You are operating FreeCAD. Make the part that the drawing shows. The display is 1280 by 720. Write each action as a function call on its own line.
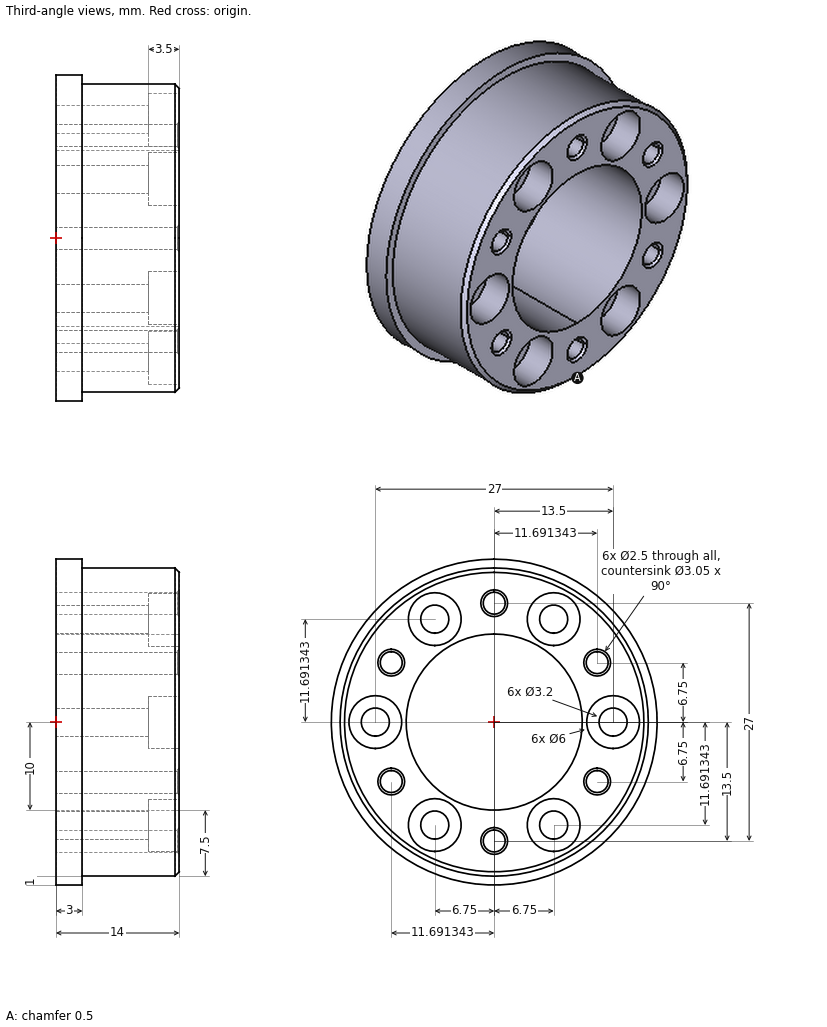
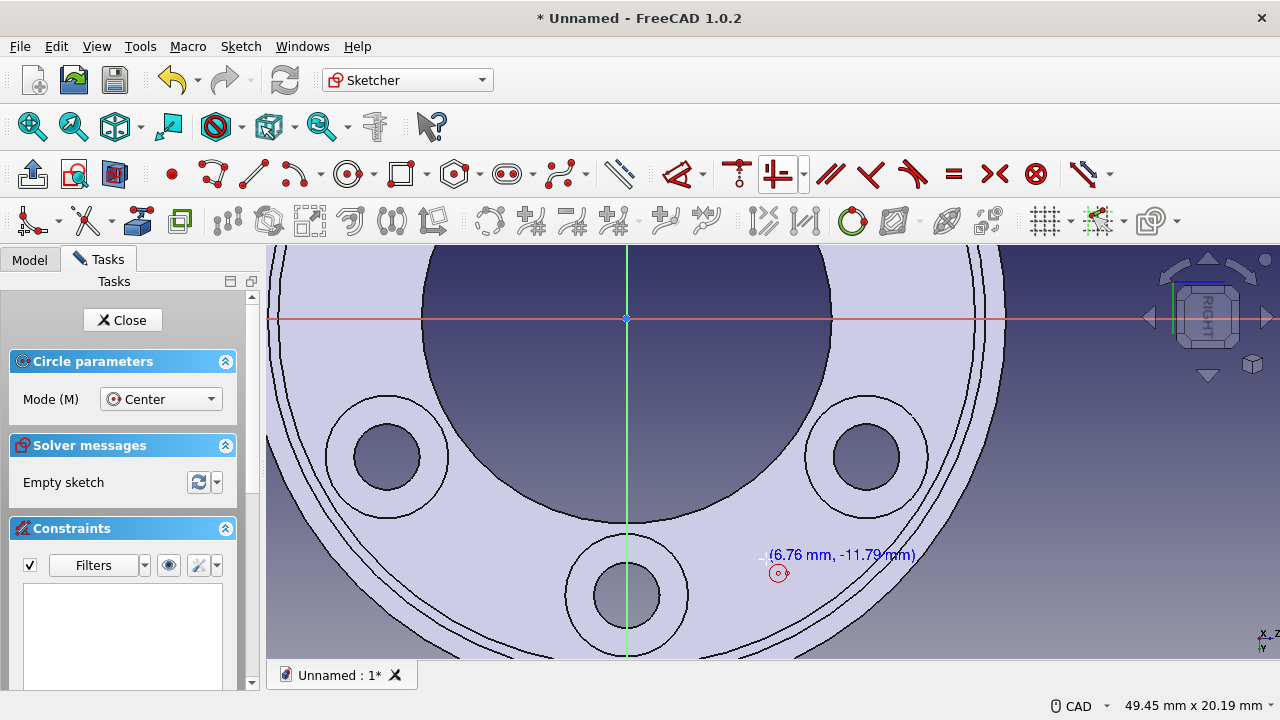
click(765, 558)
click(783, 540)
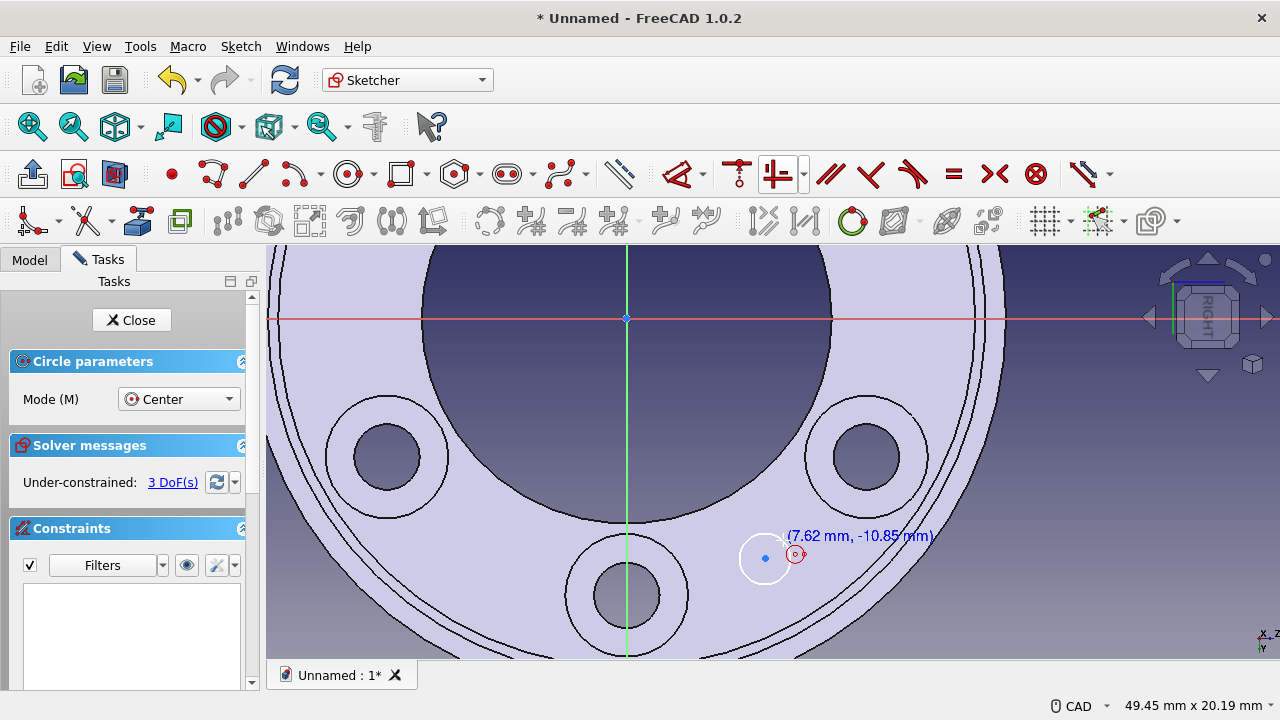
click(488, 558)
click(506, 540)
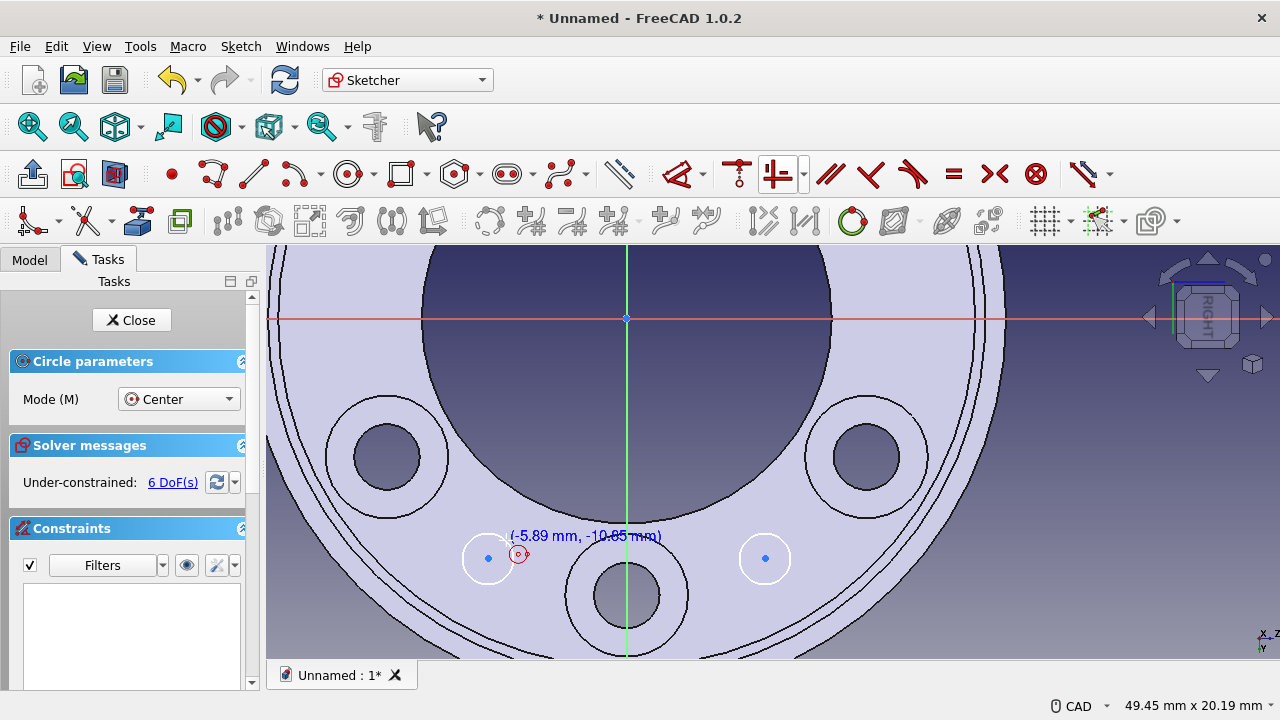
click(350, 319)
click(368, 300)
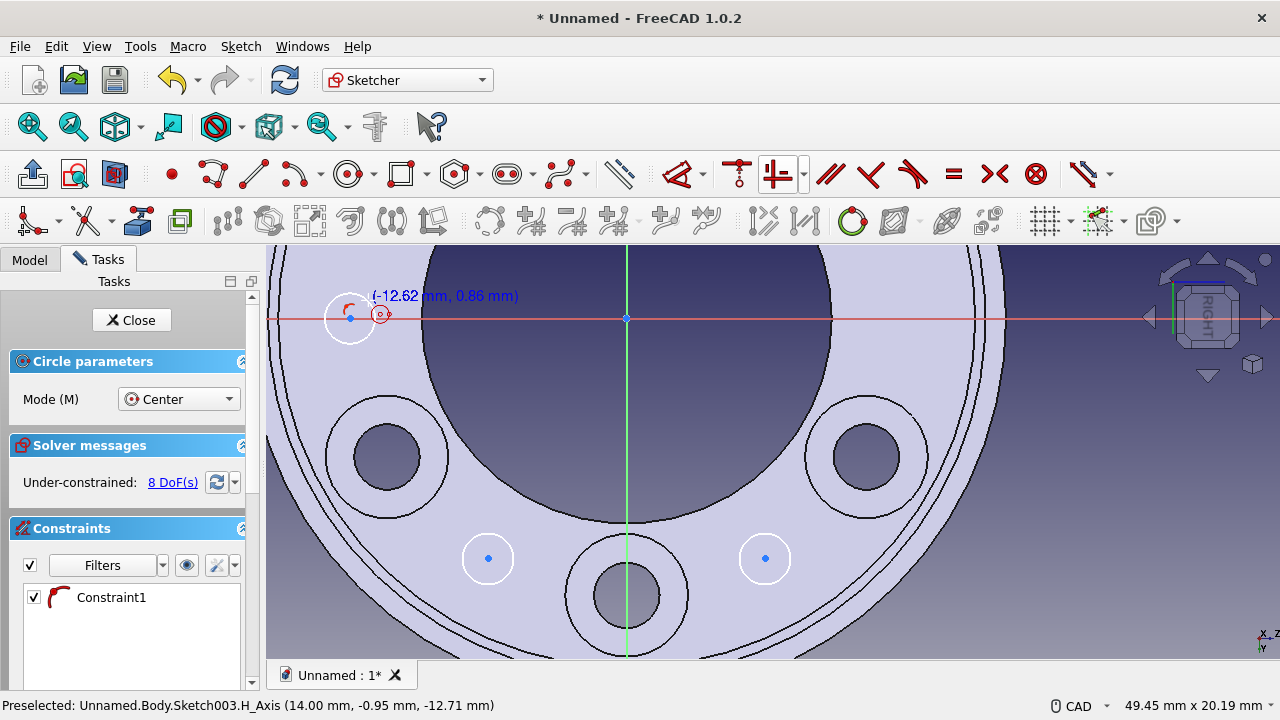
scroll(768, 561, down, 4)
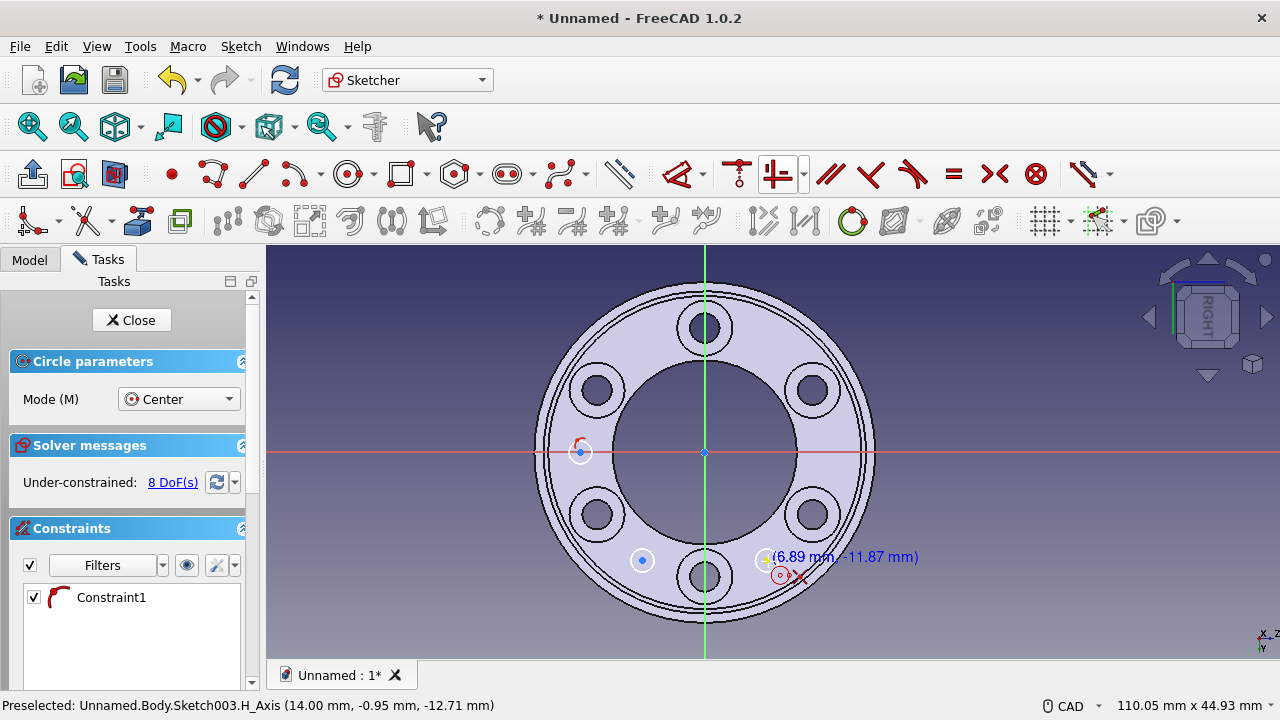
scroll(643, 345, up, 4)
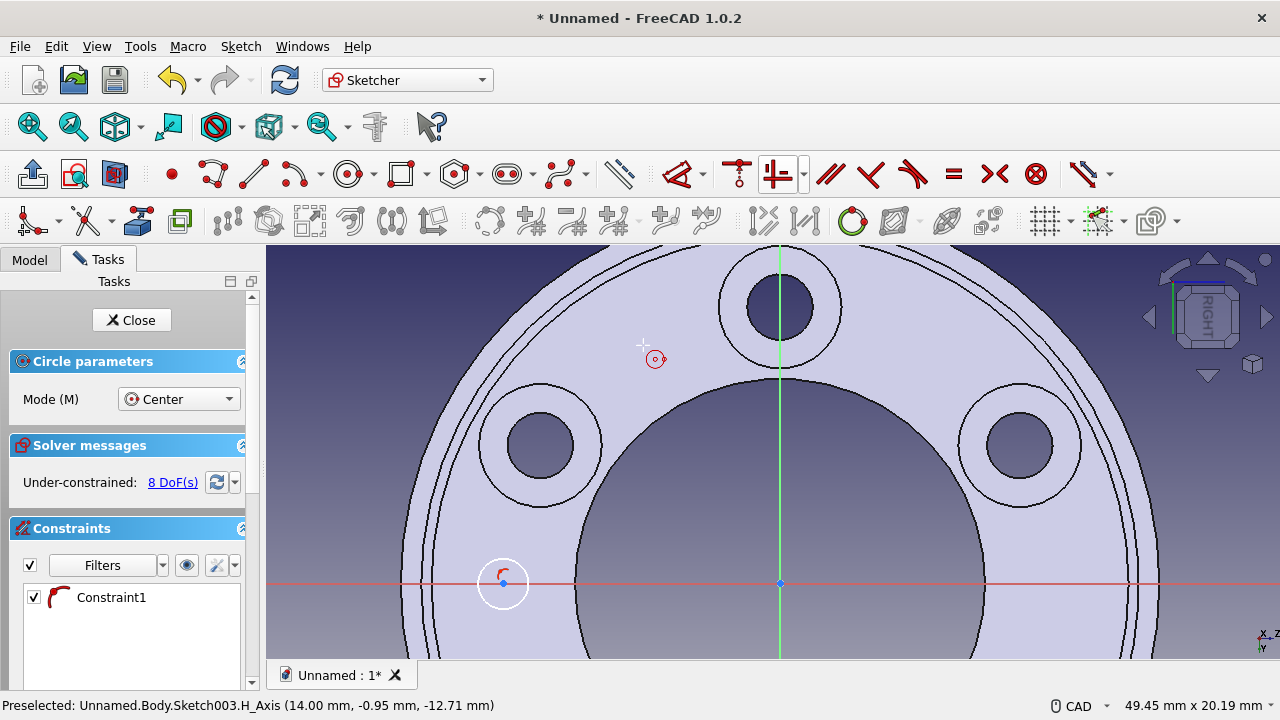
click(642, 344)
click(660, 326)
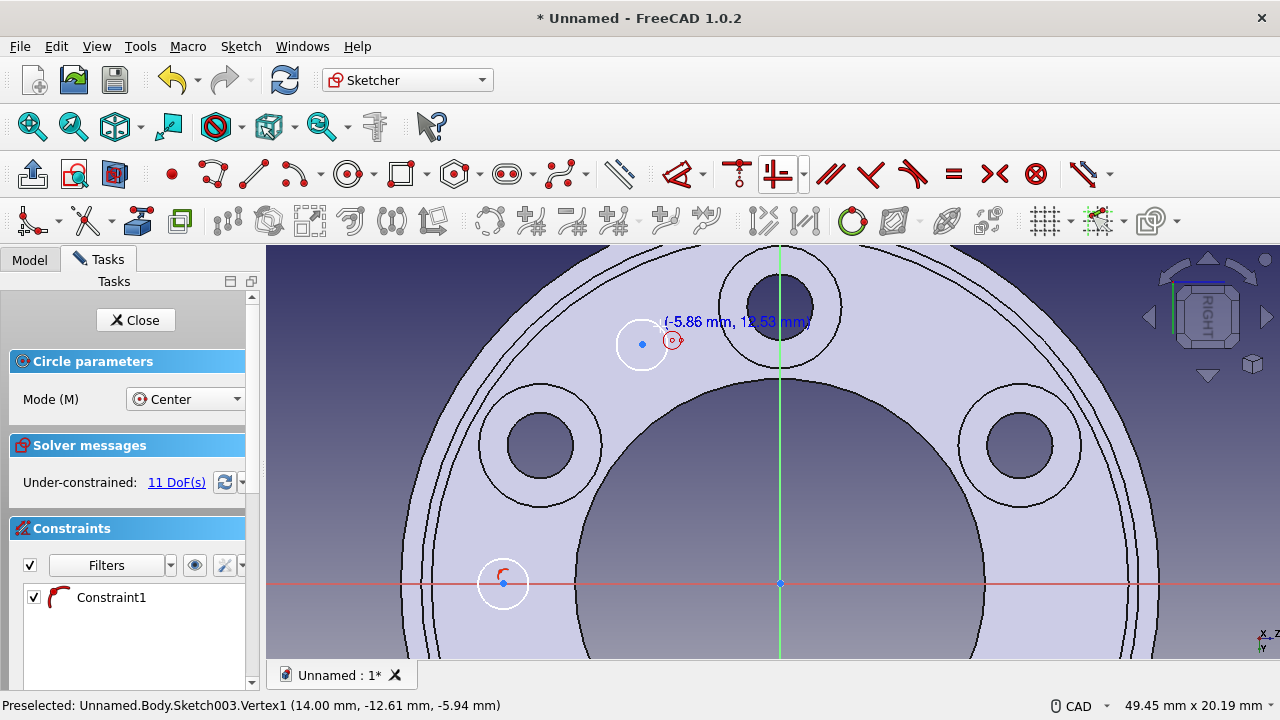
click(918, 344)
click(937, 326)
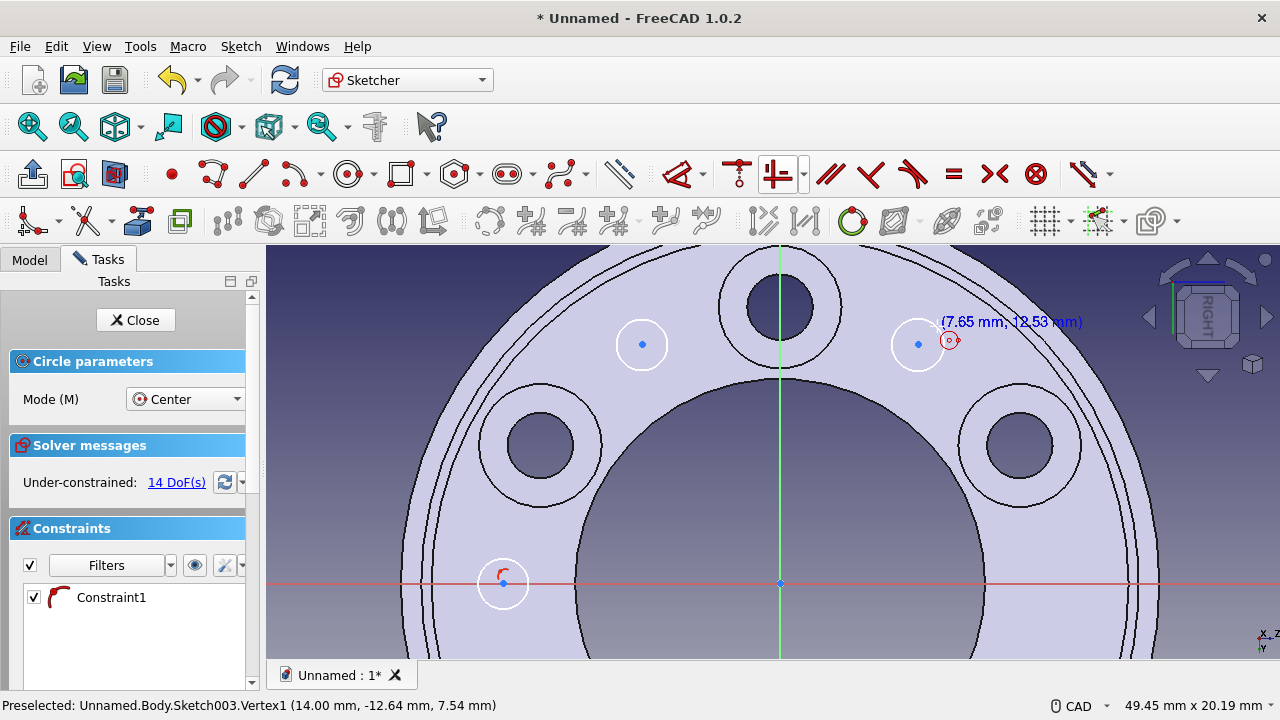
click(1057, 584)
click(1075, 566)
key(Escape)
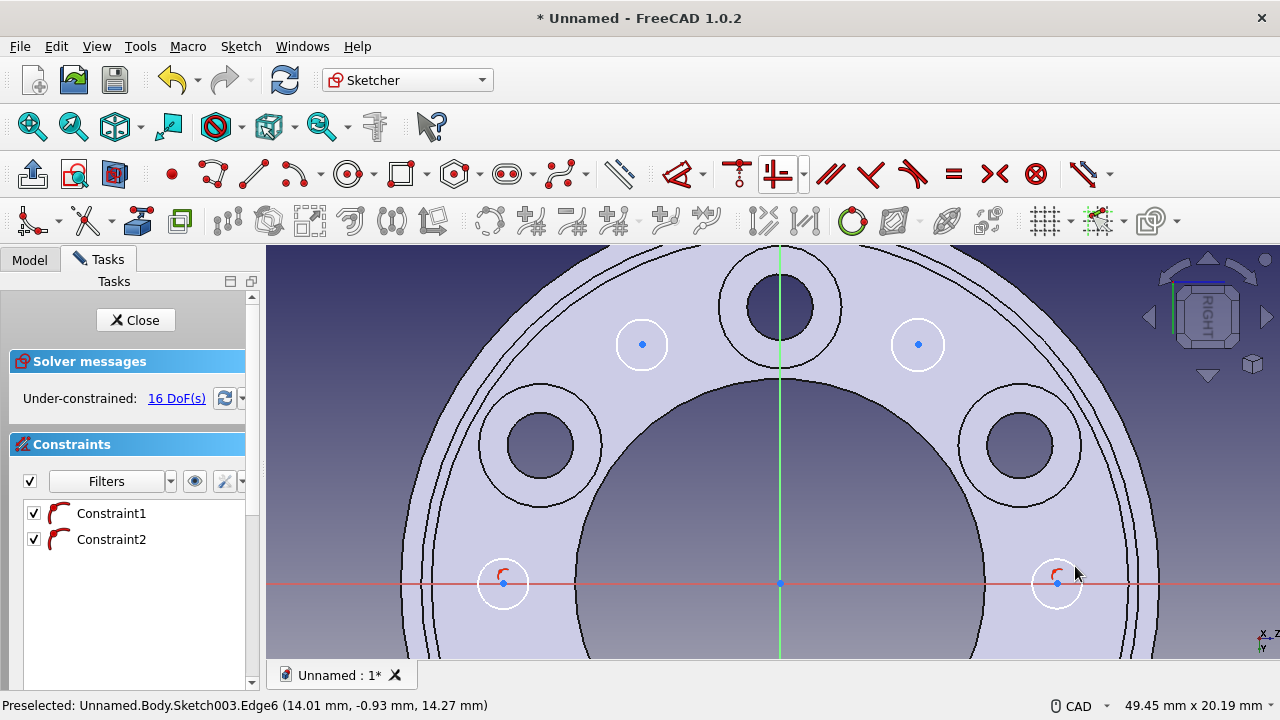
scroll(643, 344, down, 4)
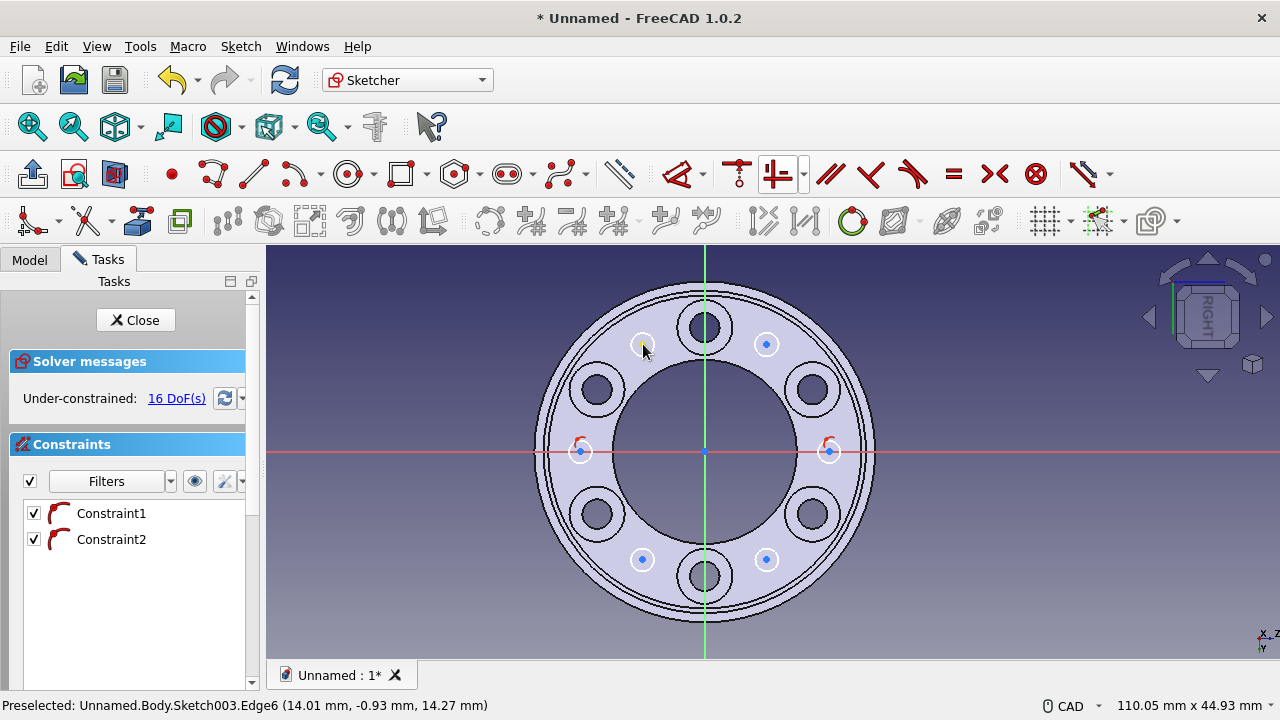
click(775, 552)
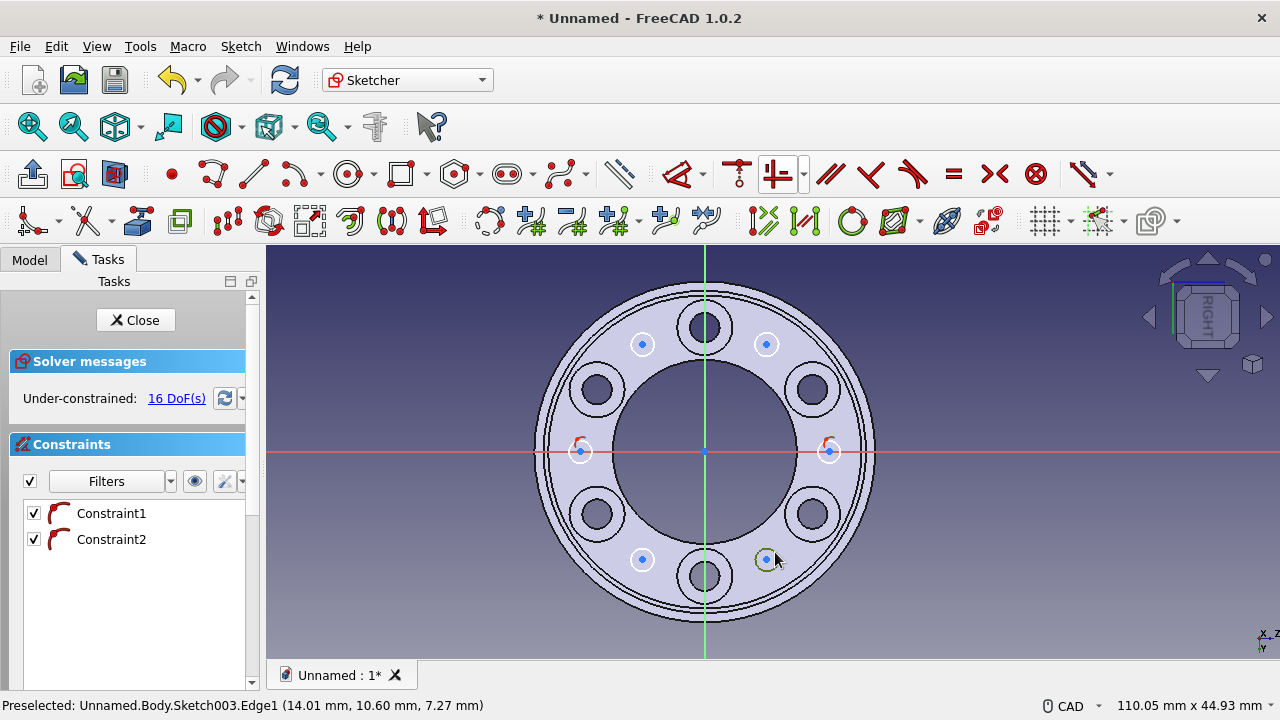
click(651, 552)